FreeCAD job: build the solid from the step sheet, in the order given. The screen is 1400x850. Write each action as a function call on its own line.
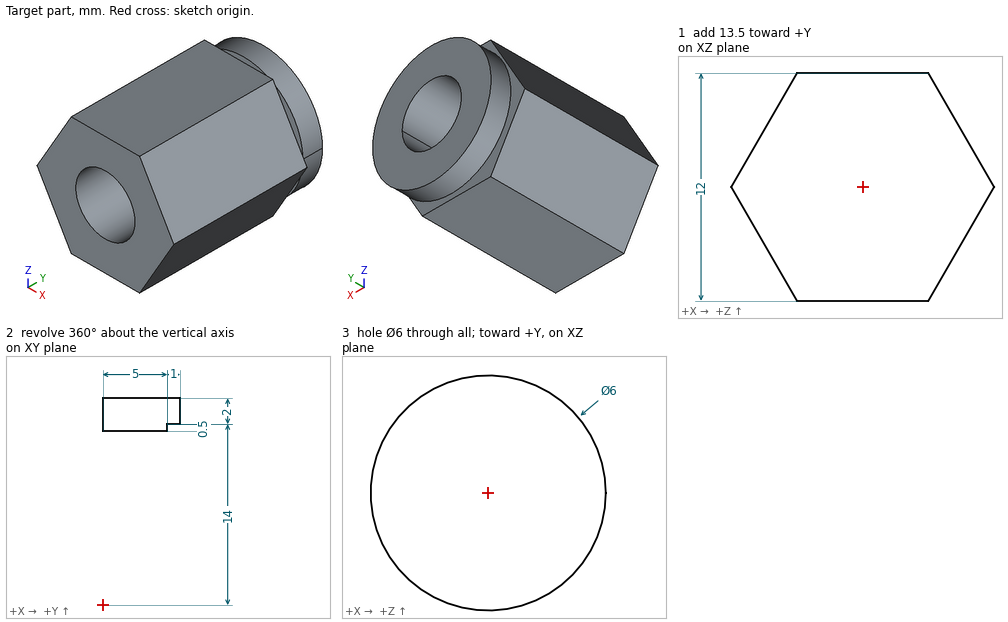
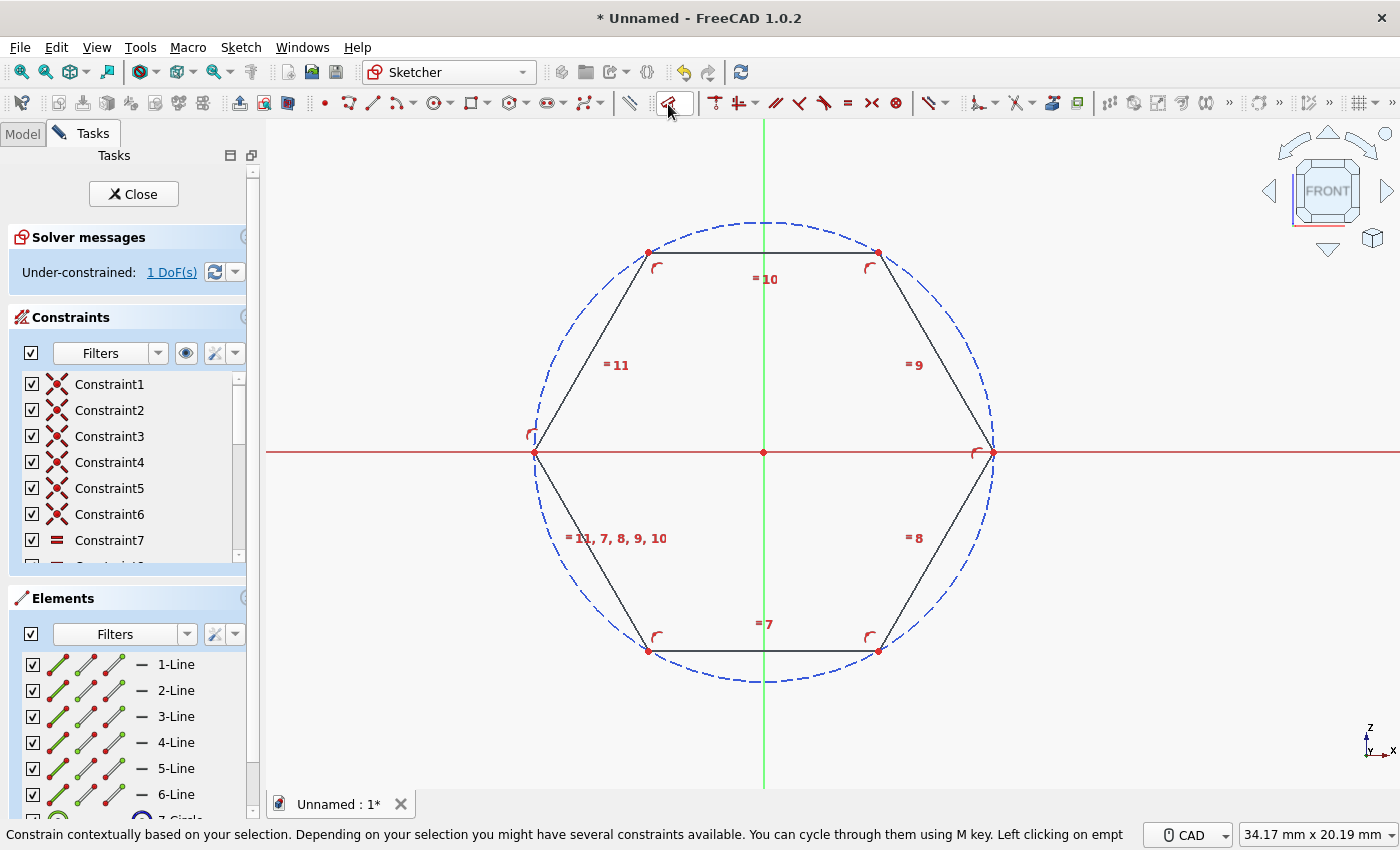
click(649, 651)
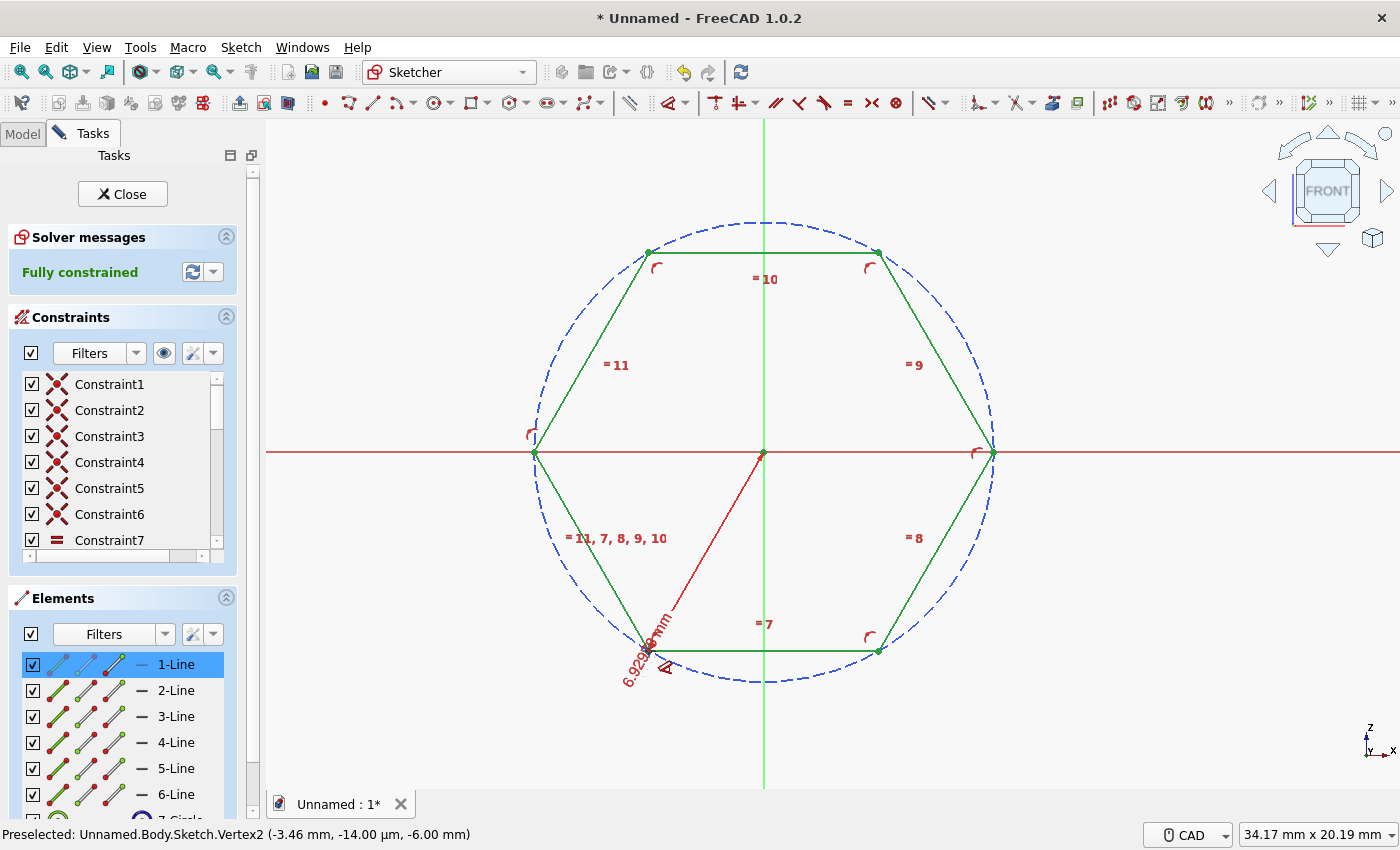
click(879, 253)
click(913, 360)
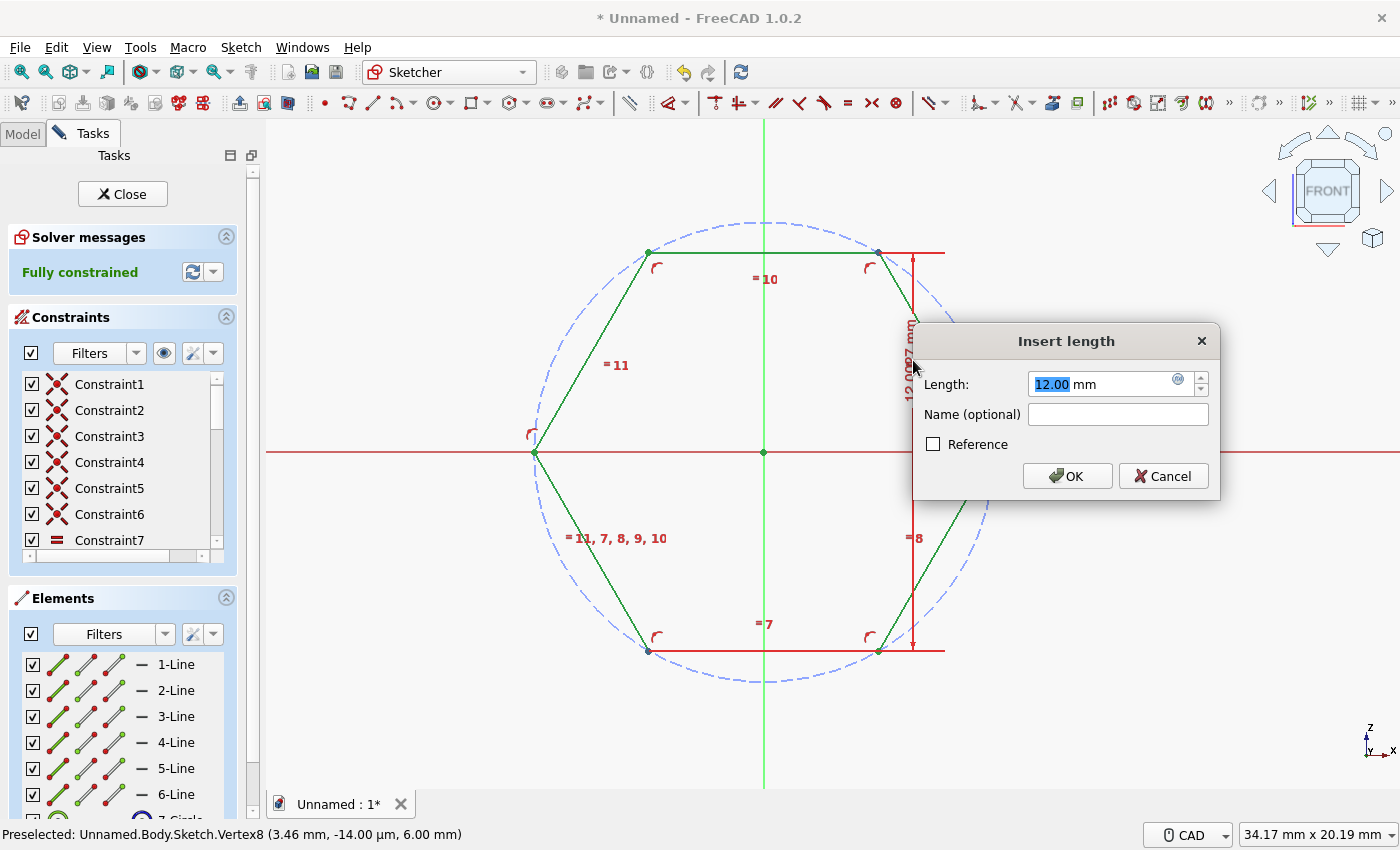
text(12)
key(Return)
key(Escape)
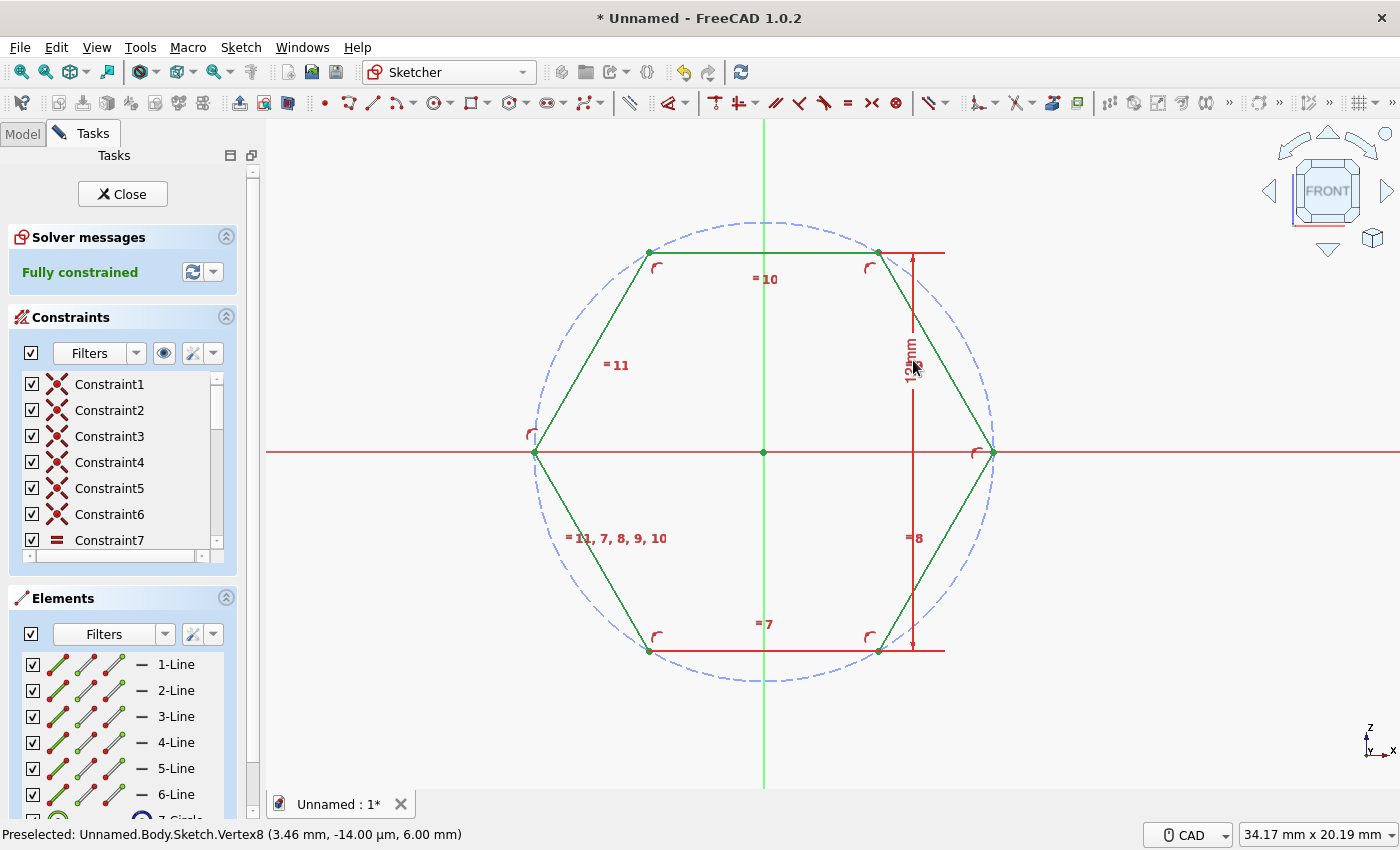
click(123, 194)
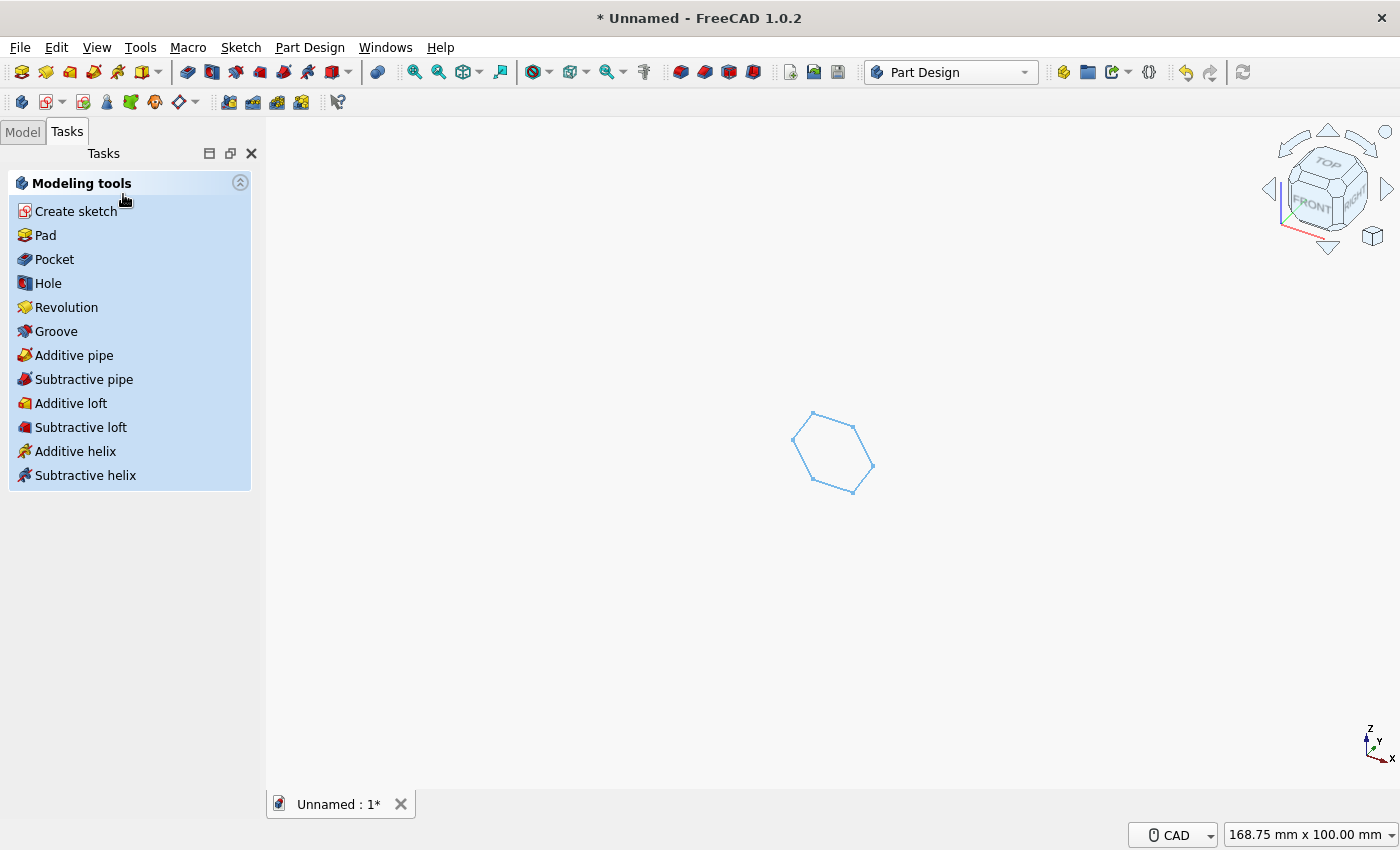
click(22, 72)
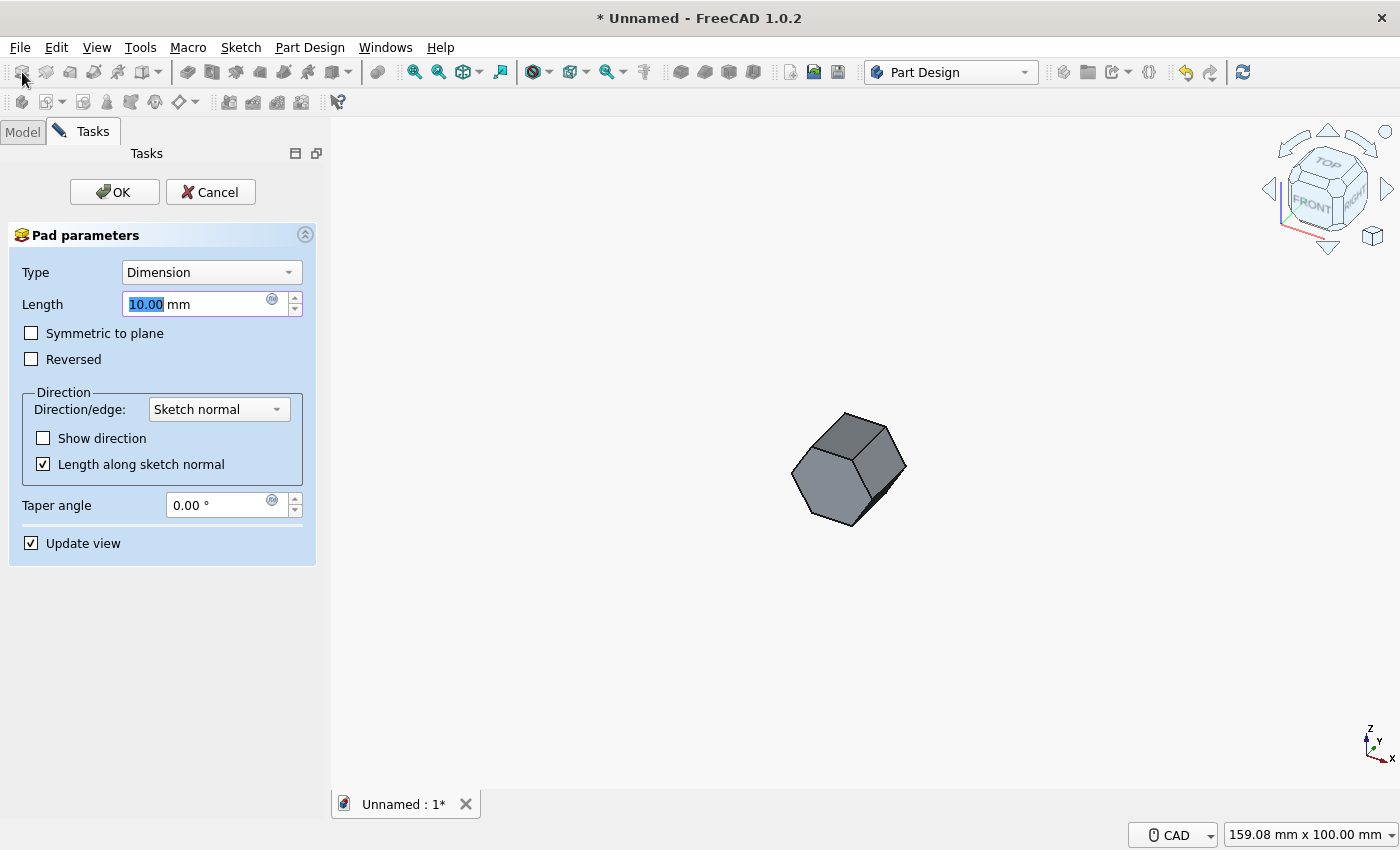
text(13.5)
key(Tab)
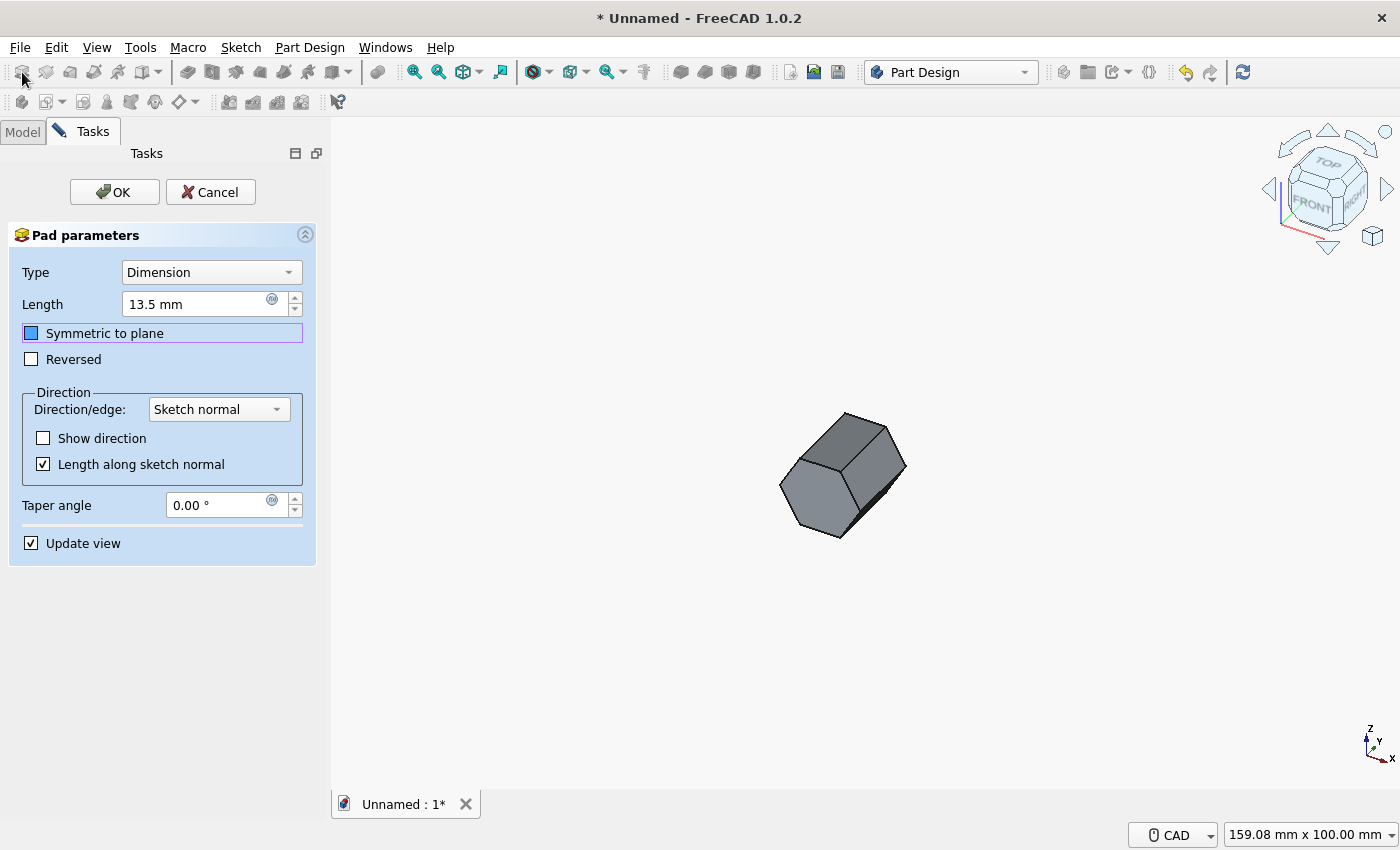
click(30, 359)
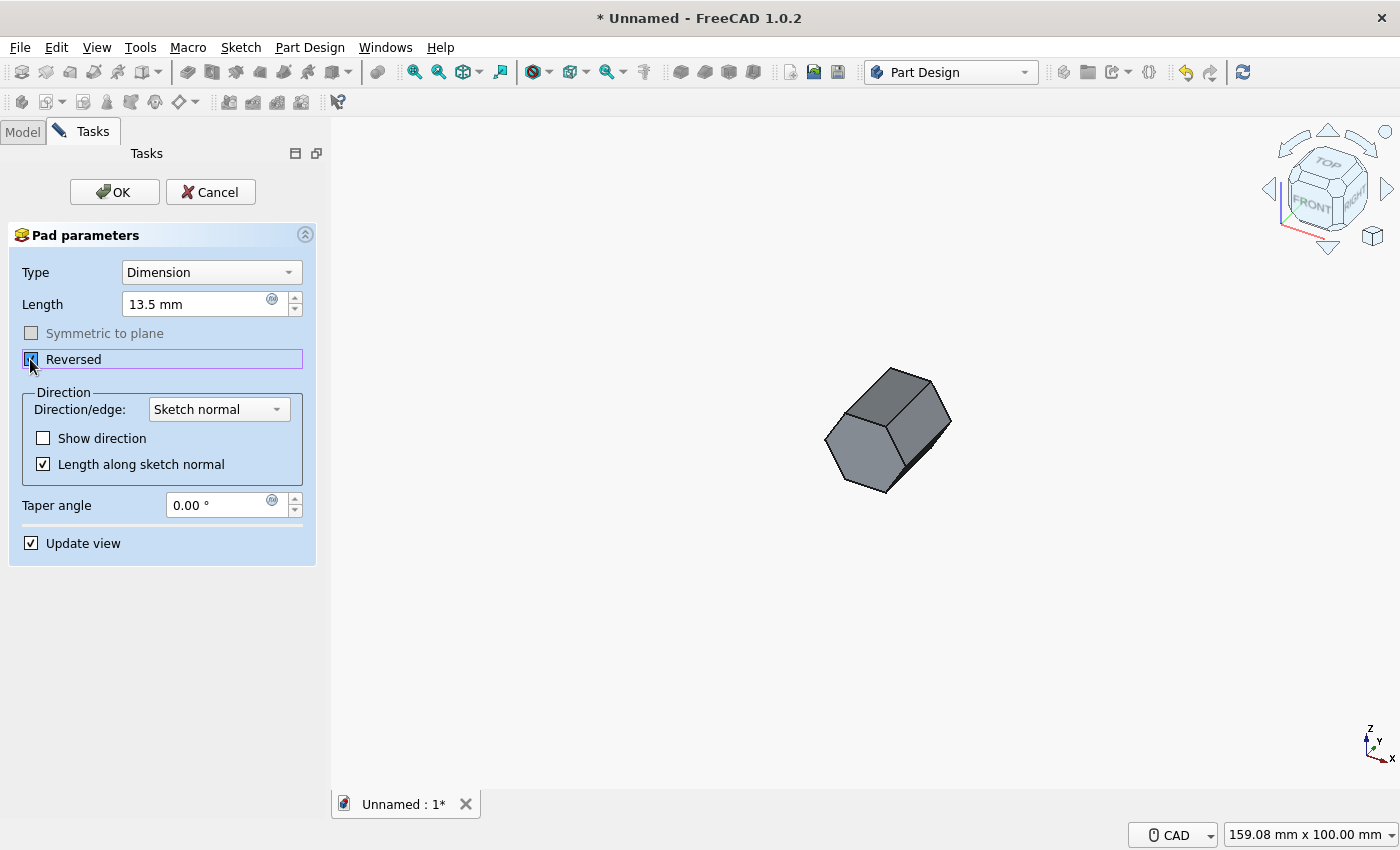
click(115, 192)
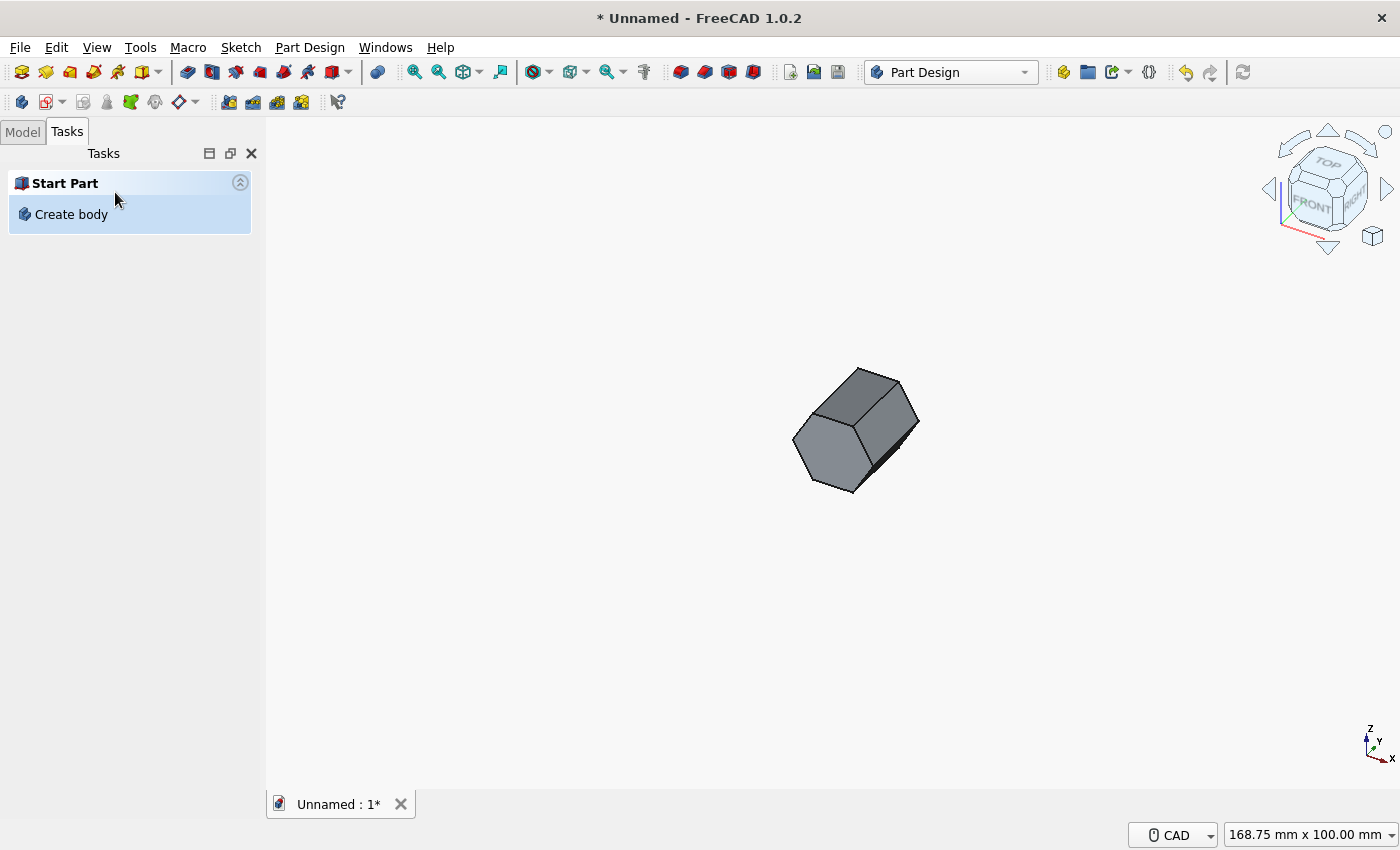
click(416, 72)